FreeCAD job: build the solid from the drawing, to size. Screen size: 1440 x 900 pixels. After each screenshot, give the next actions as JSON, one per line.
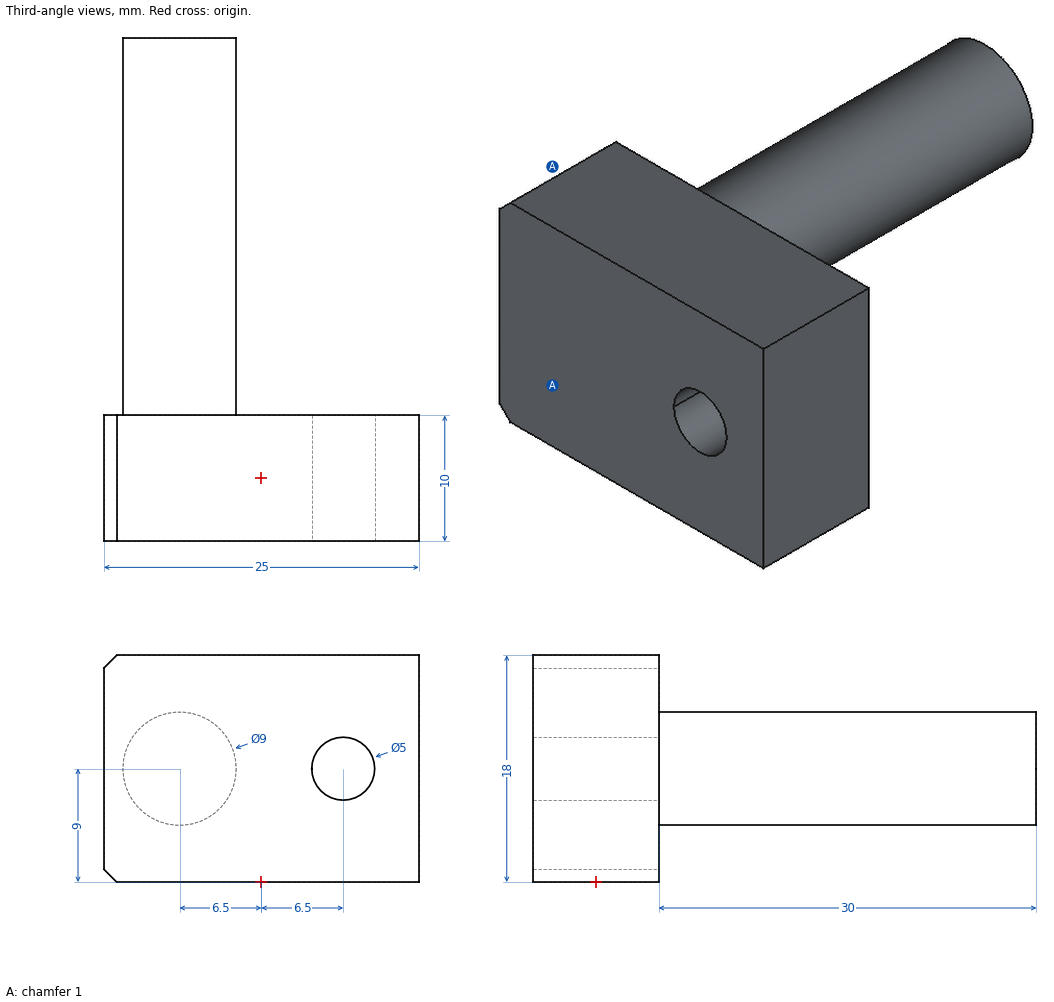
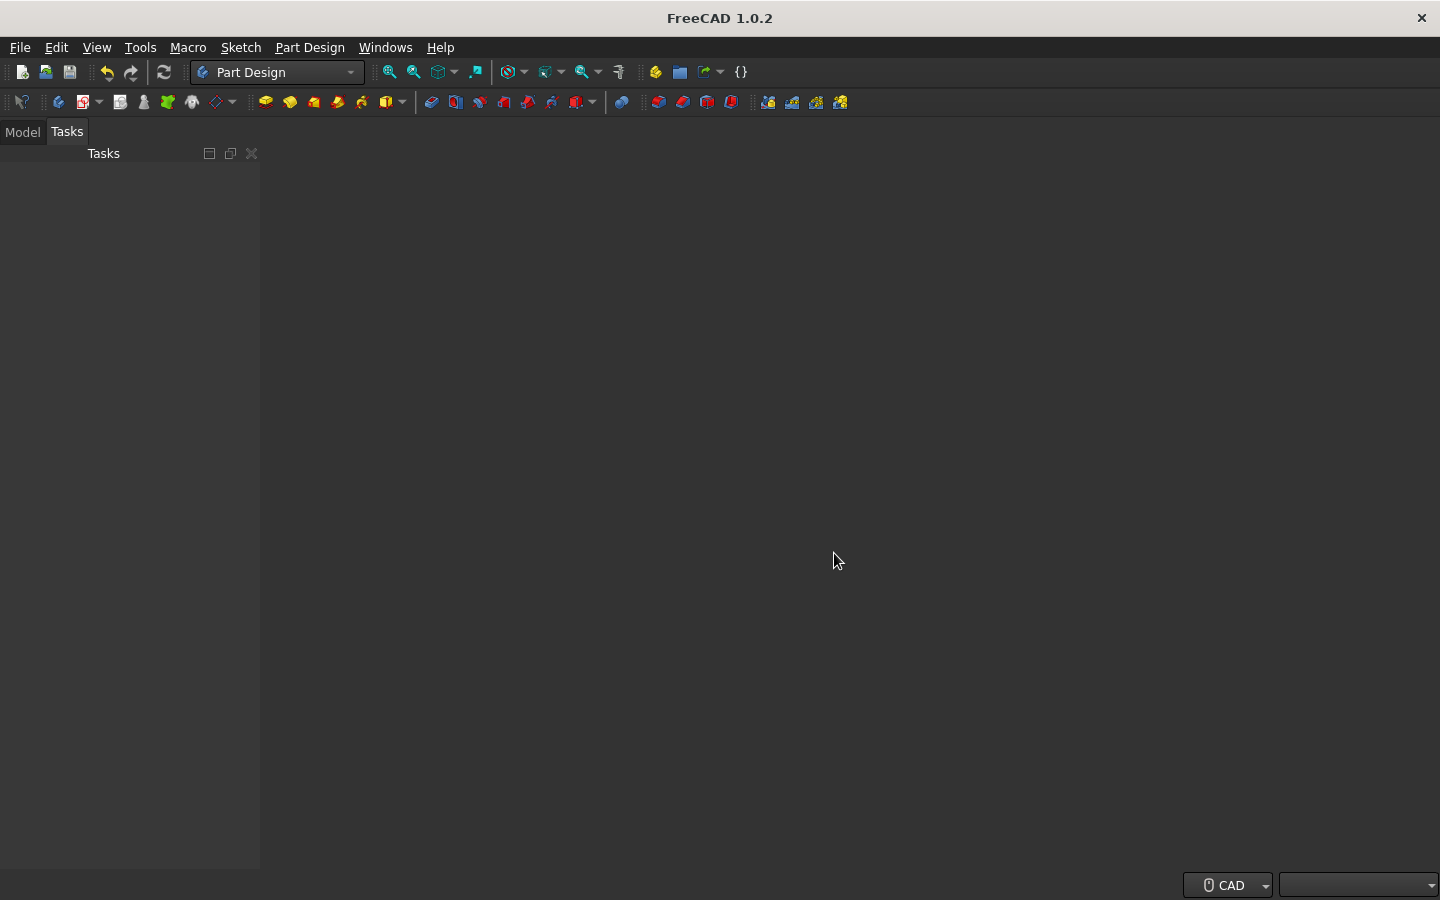
{"action": "left_click", "coordinate": [22, 72]}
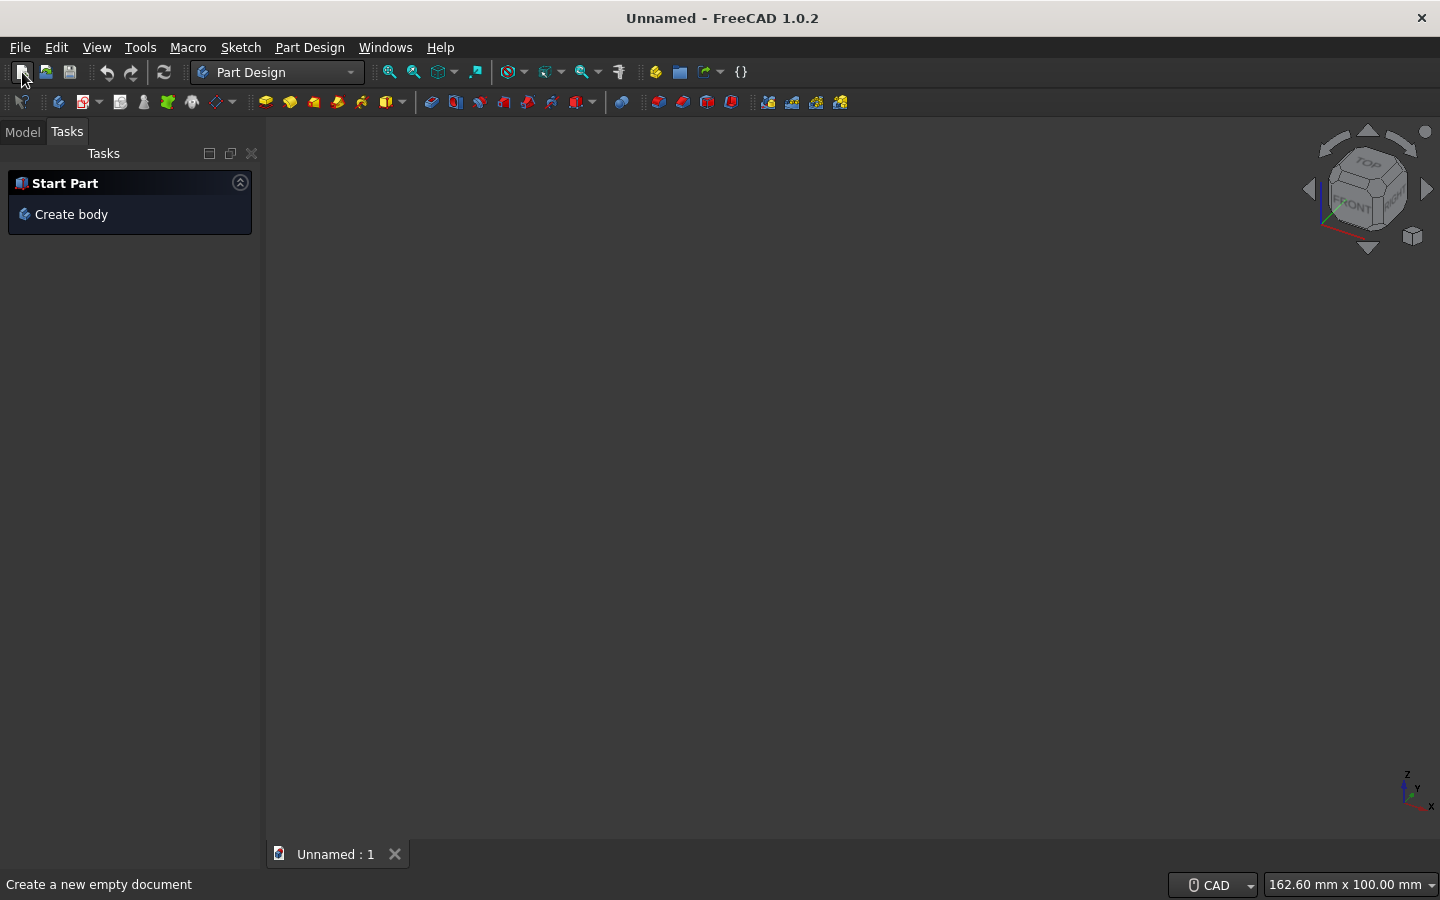
{"action": "left_click", "coordinate": [84, 102]}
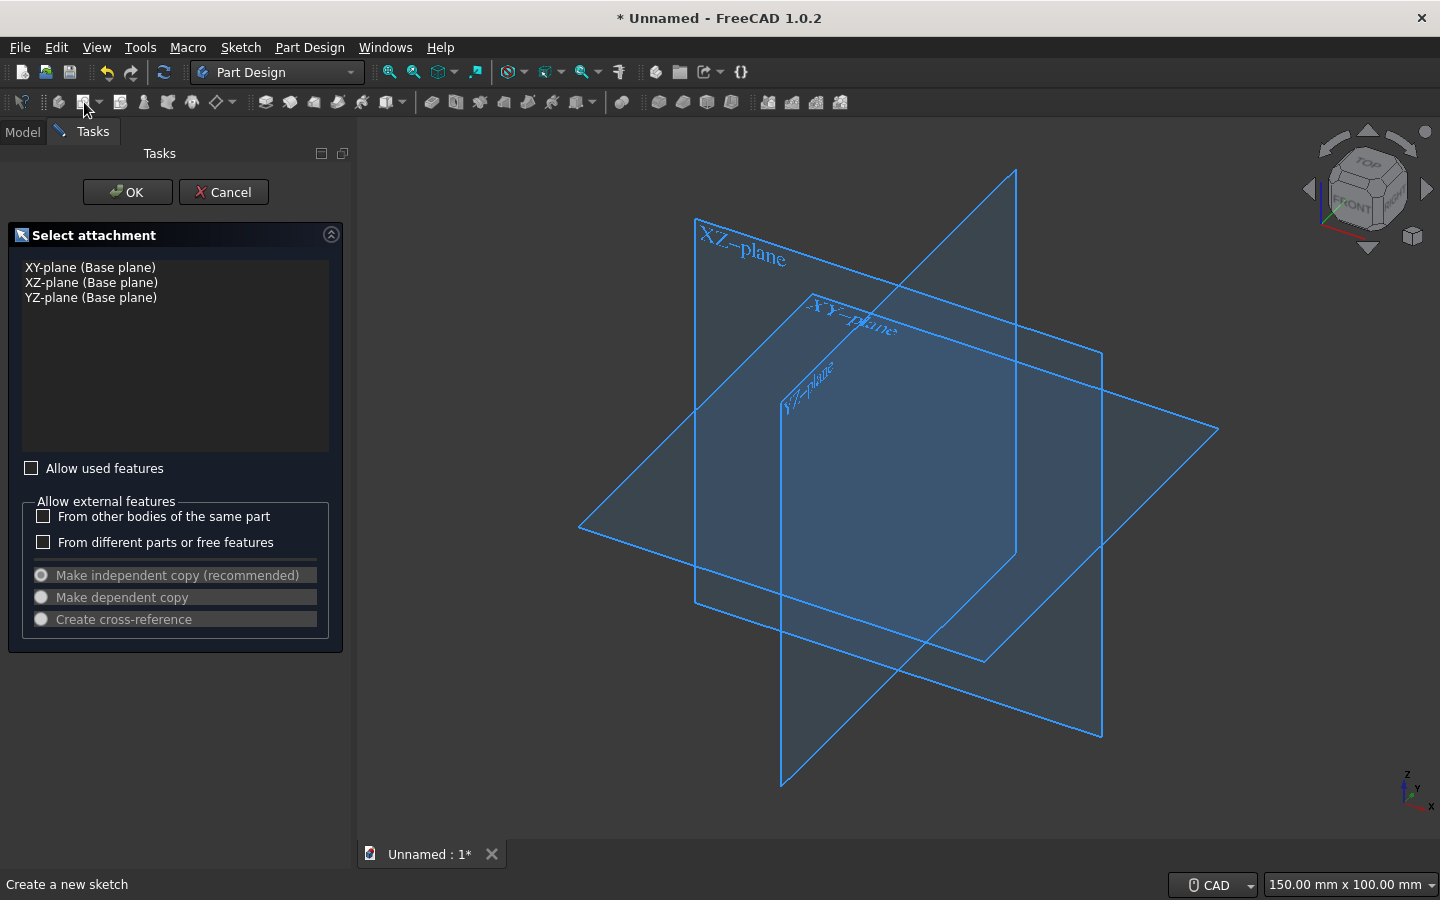
{"action": "left_click", "coordinate": [82, 268]}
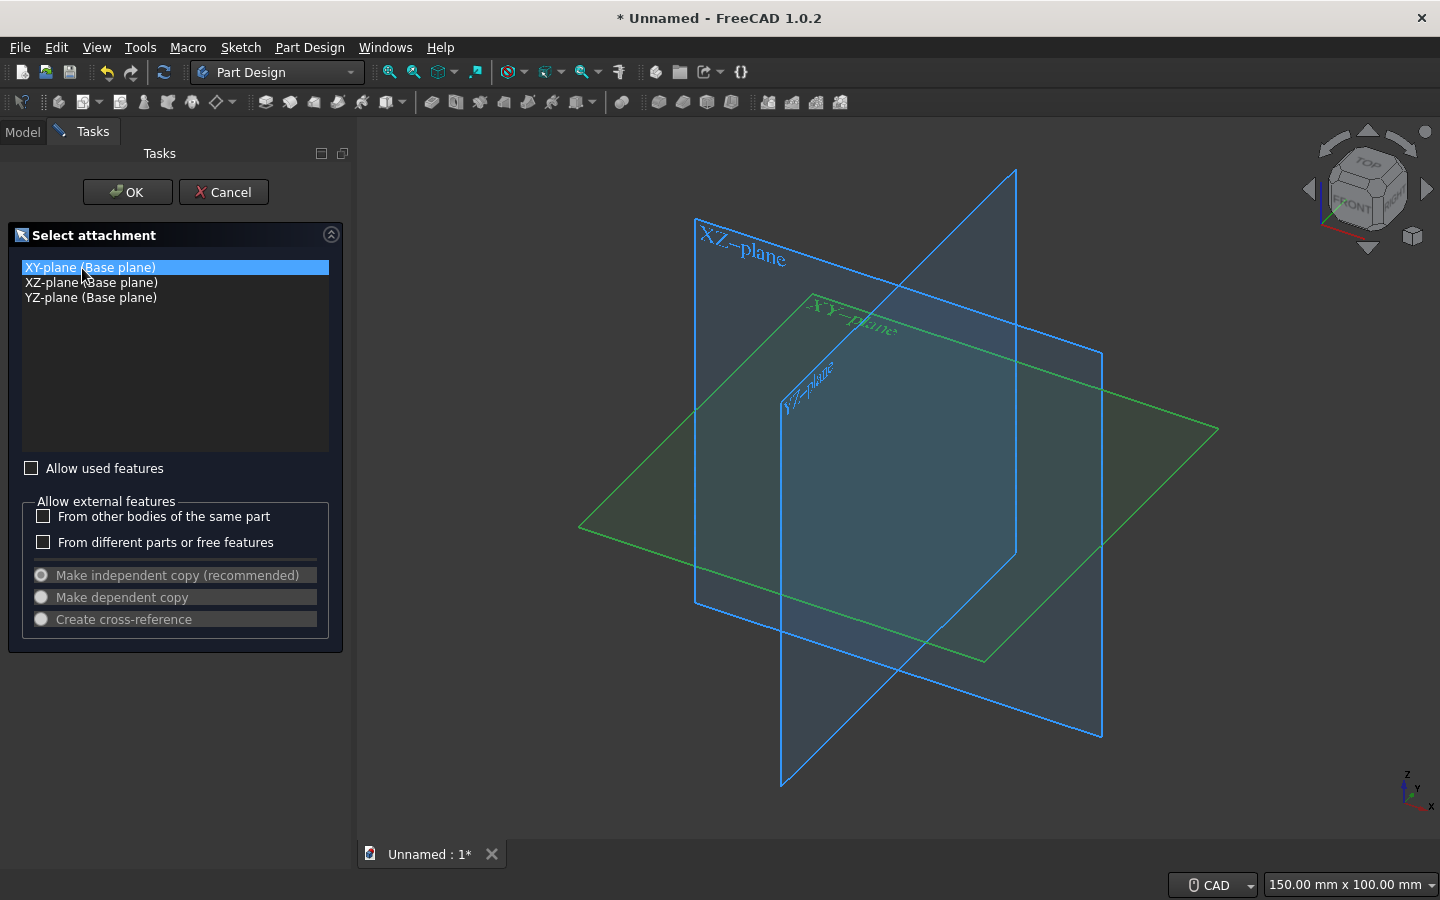
{"action": "left_click", "coordinate": [128, 192]}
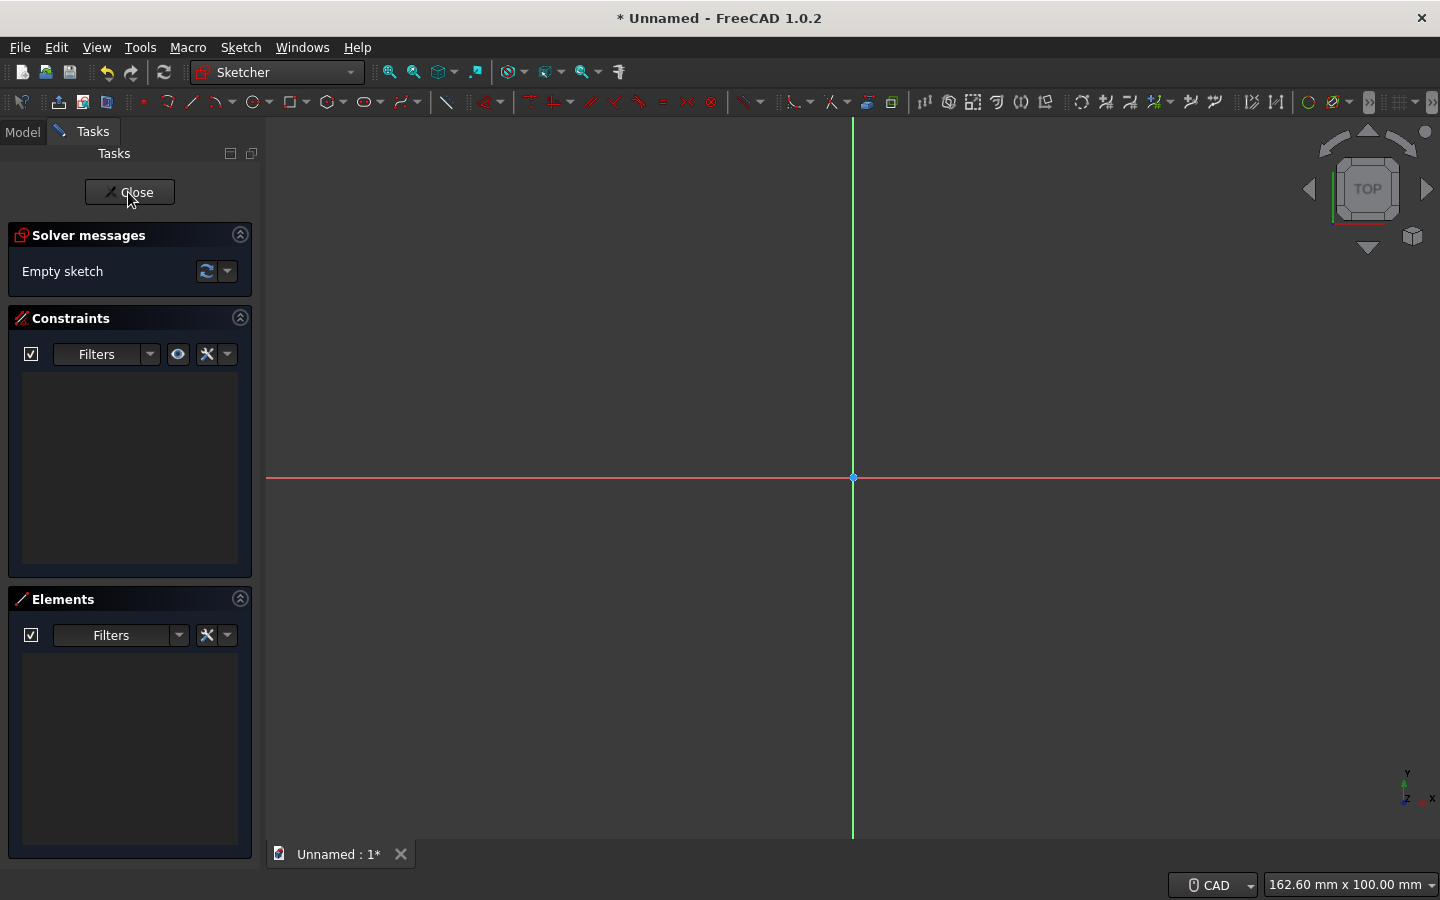
{"action": "scroll", "coordinate": [875, 478], "scroll_direction": "up", "scroll_amount": 7}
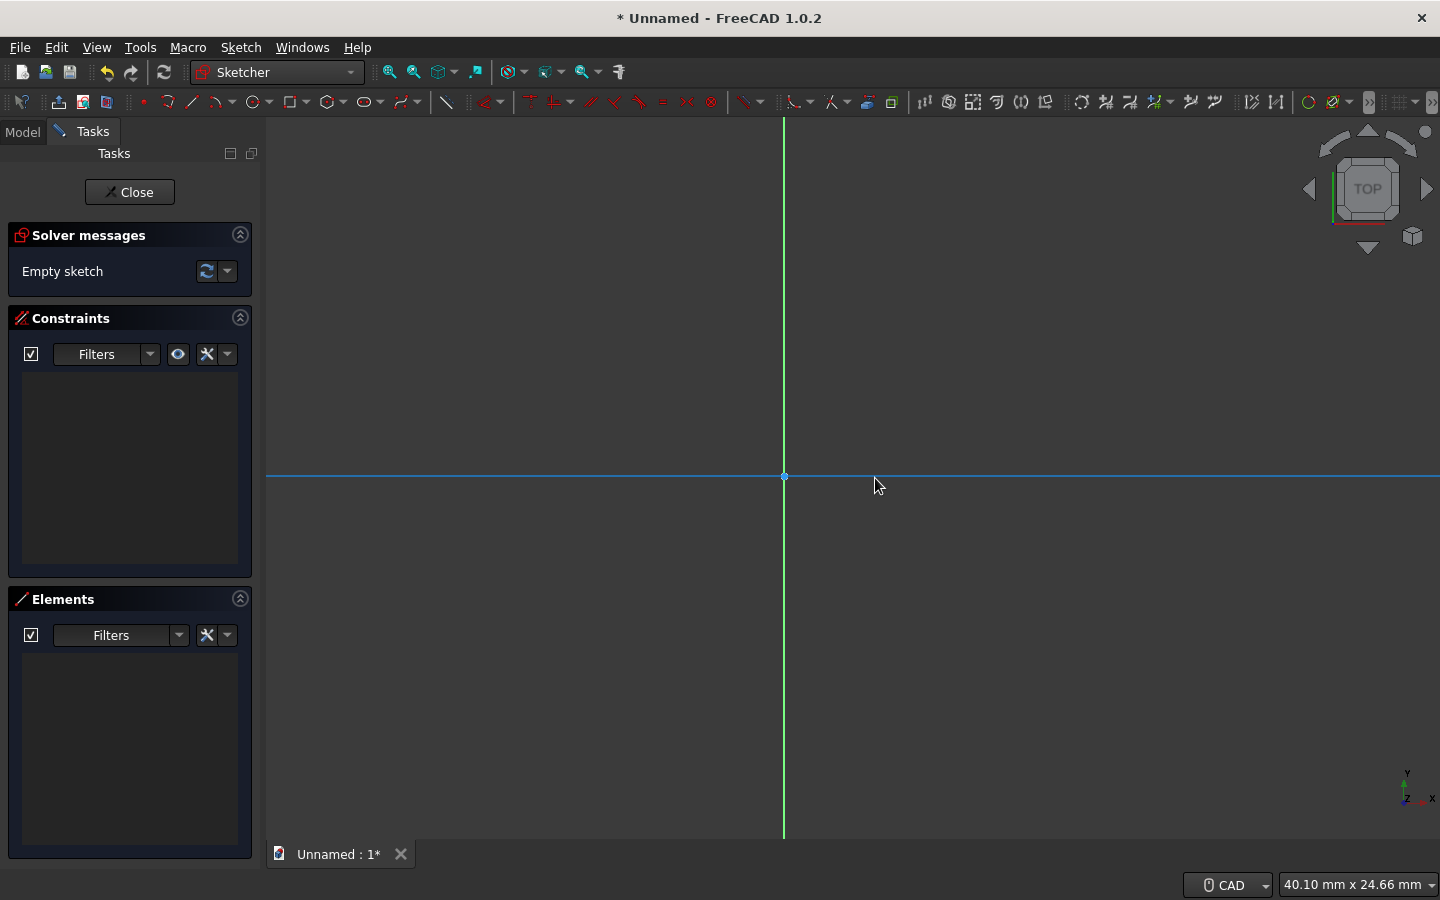
{"action": "left_click", "coordinate": [308, 102]}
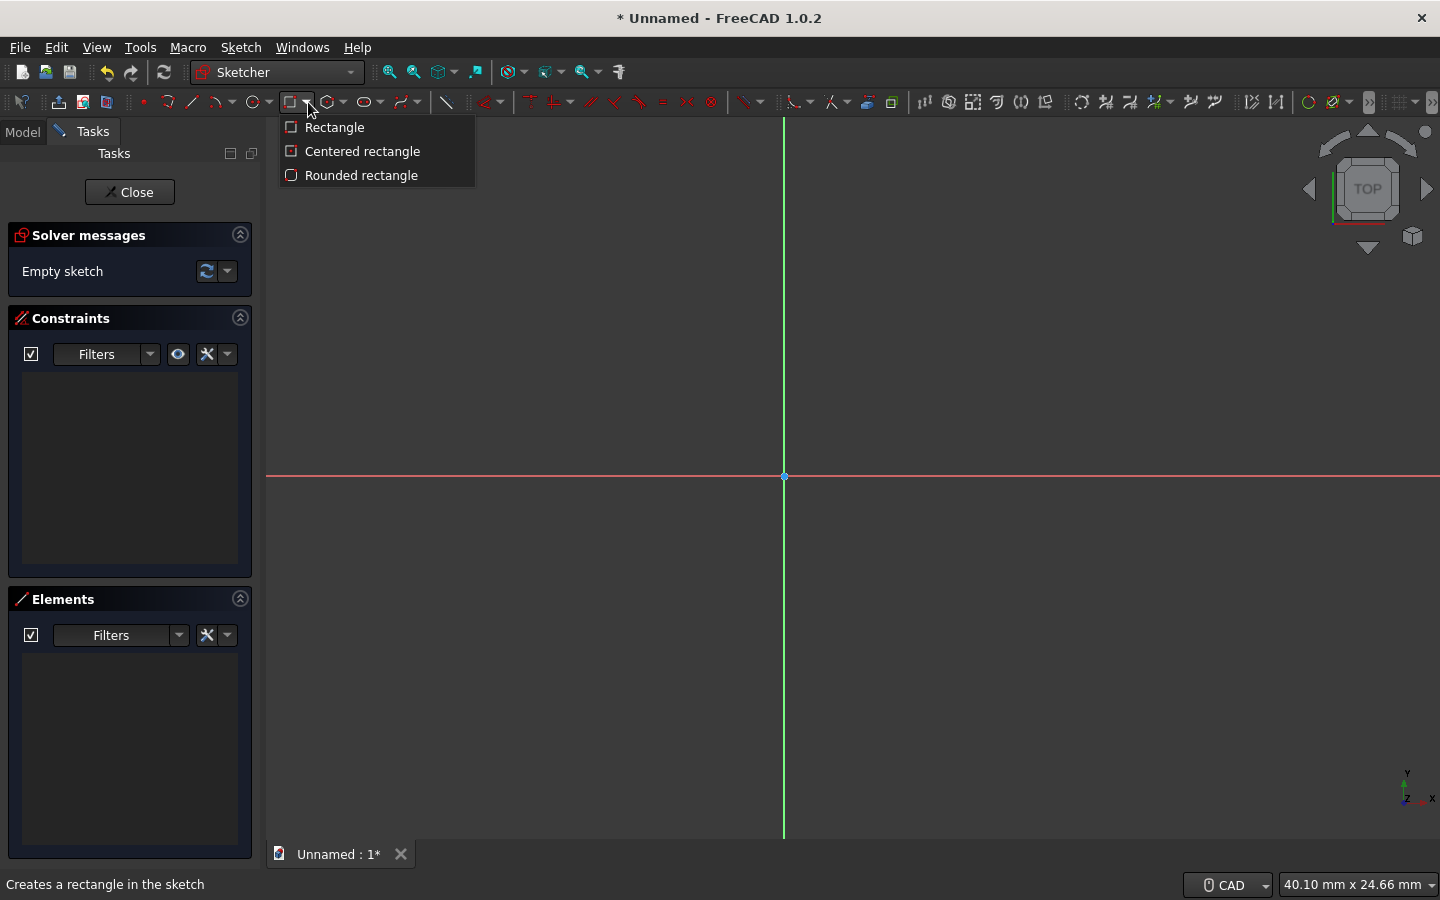
{"action": "left_click", "coordinate": [378, 151]}